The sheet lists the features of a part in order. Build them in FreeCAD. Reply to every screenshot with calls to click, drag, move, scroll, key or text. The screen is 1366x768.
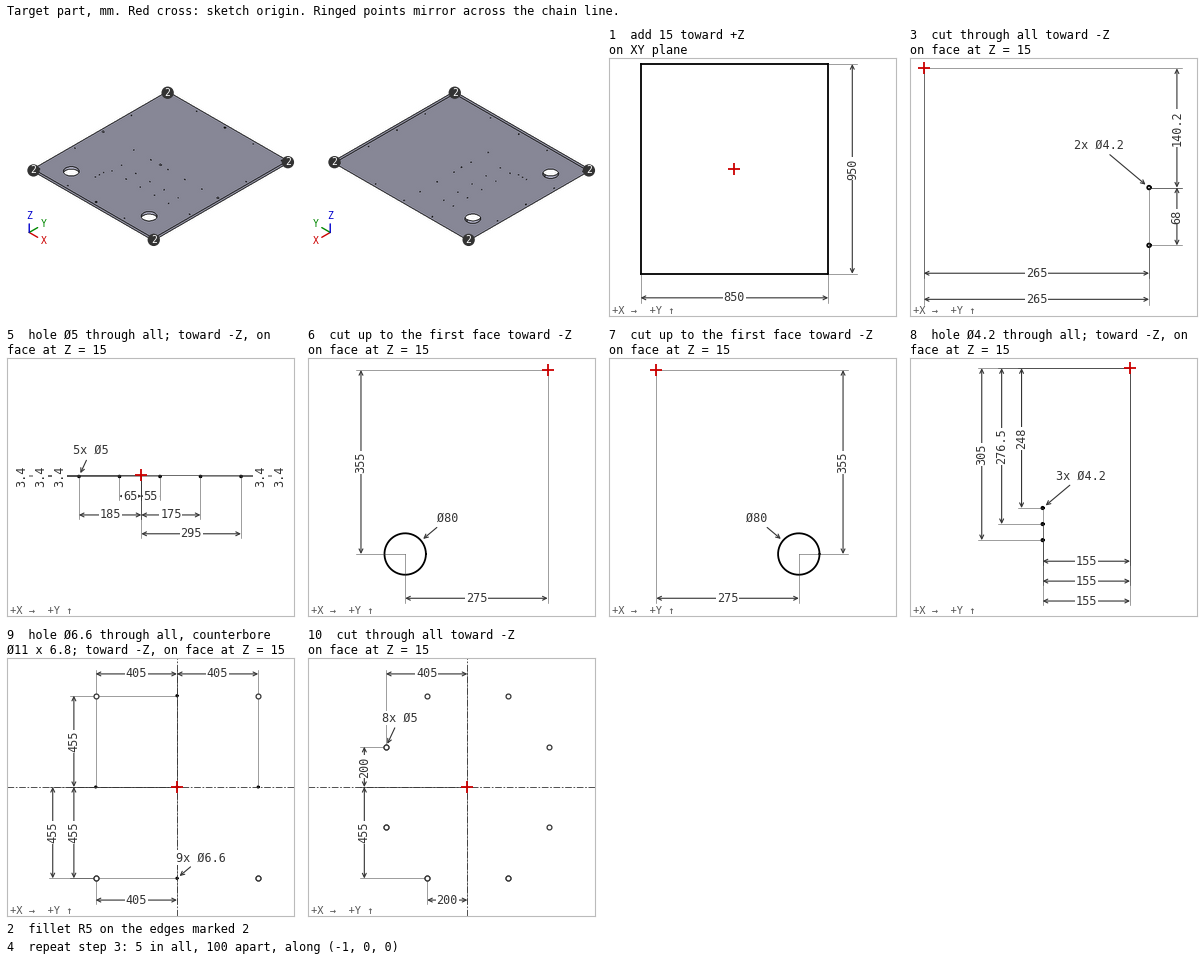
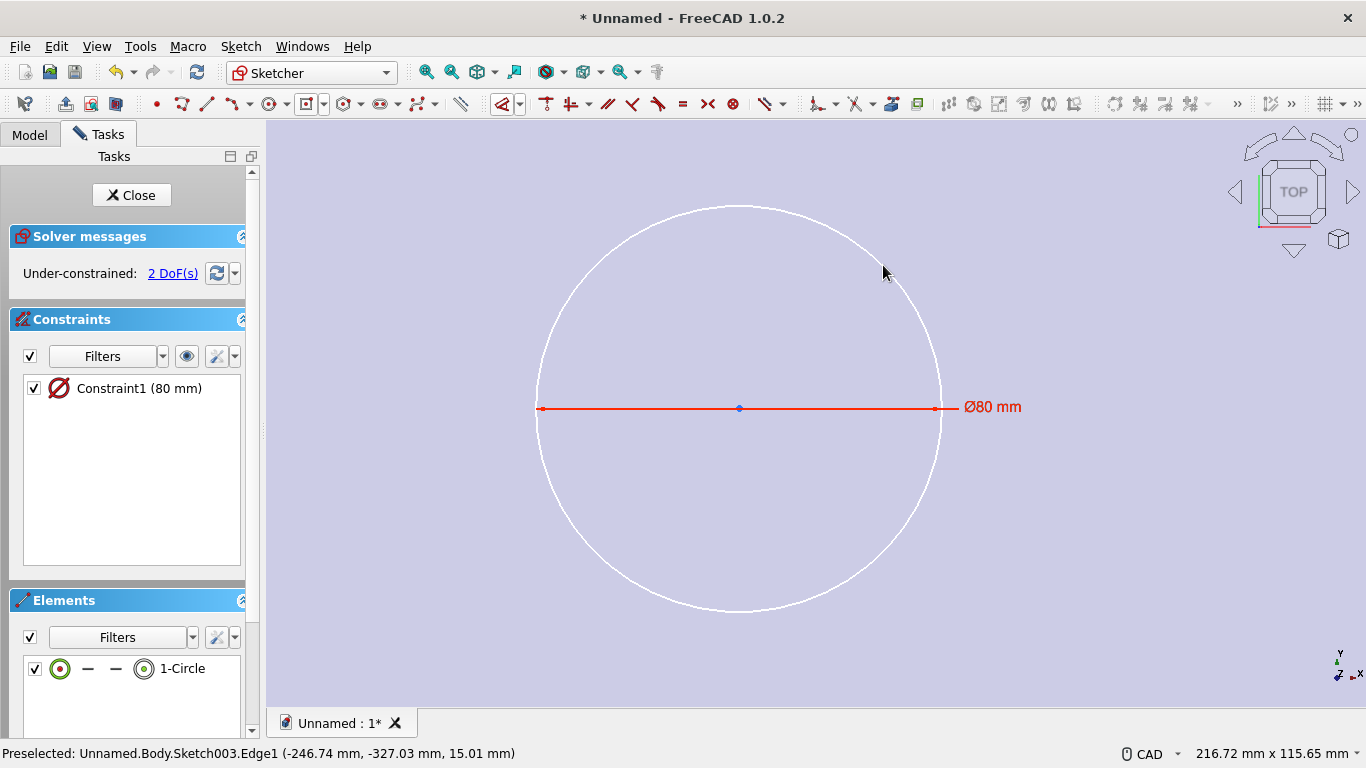
click(739, 409)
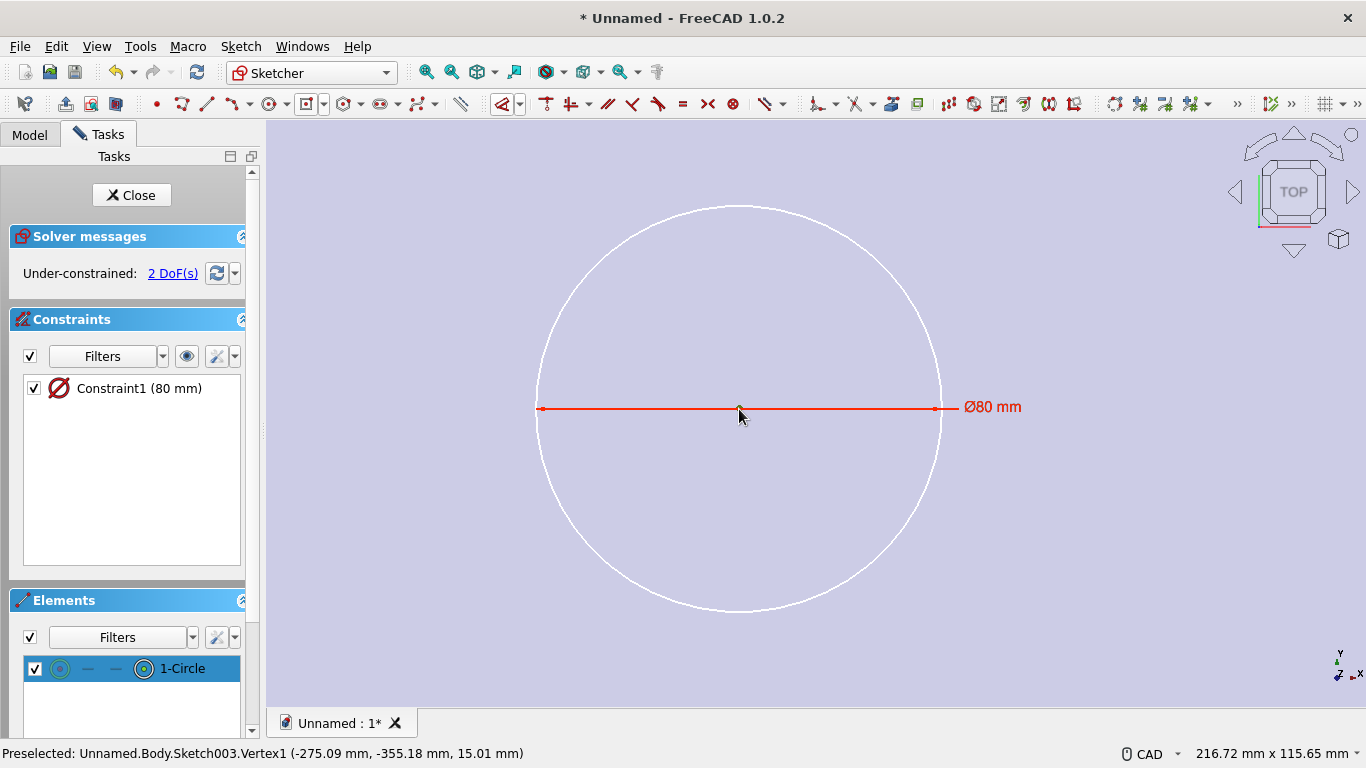
click(520, 104)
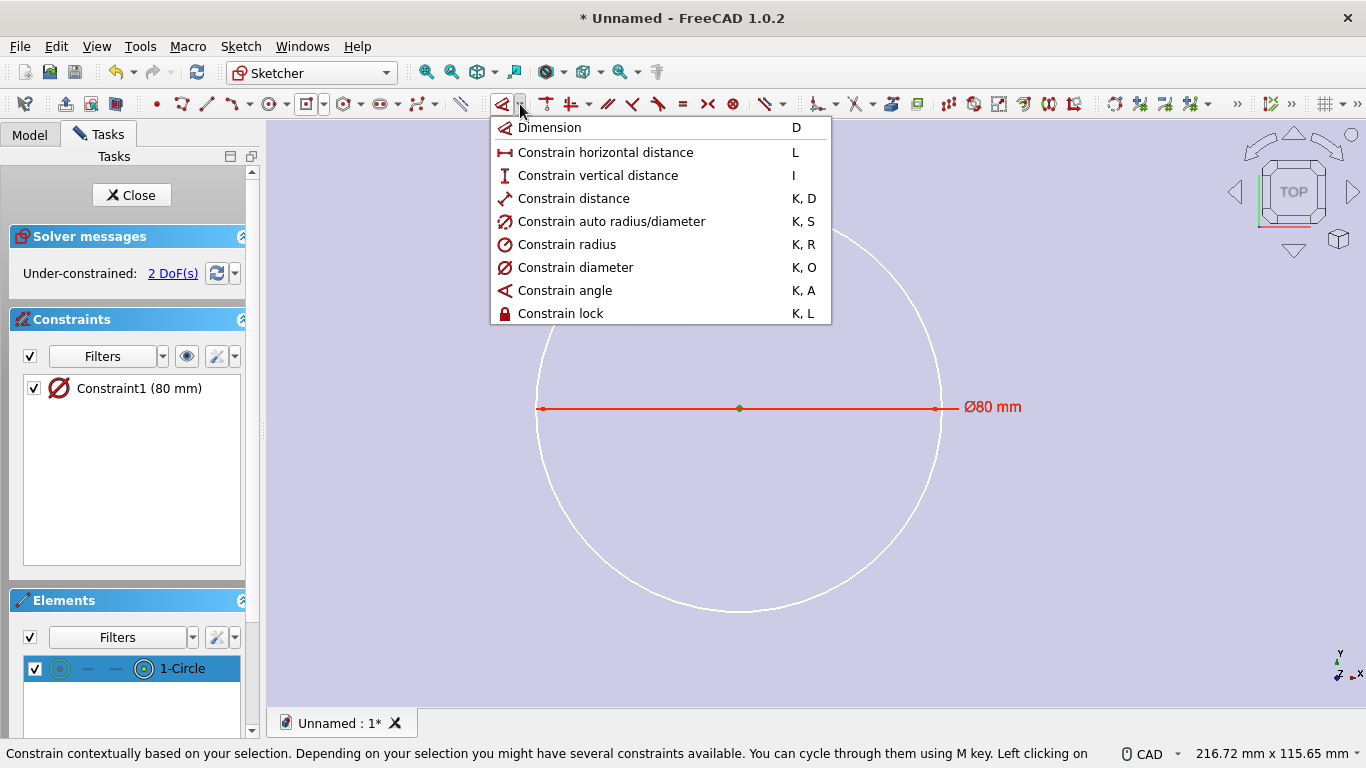
click(661, 152)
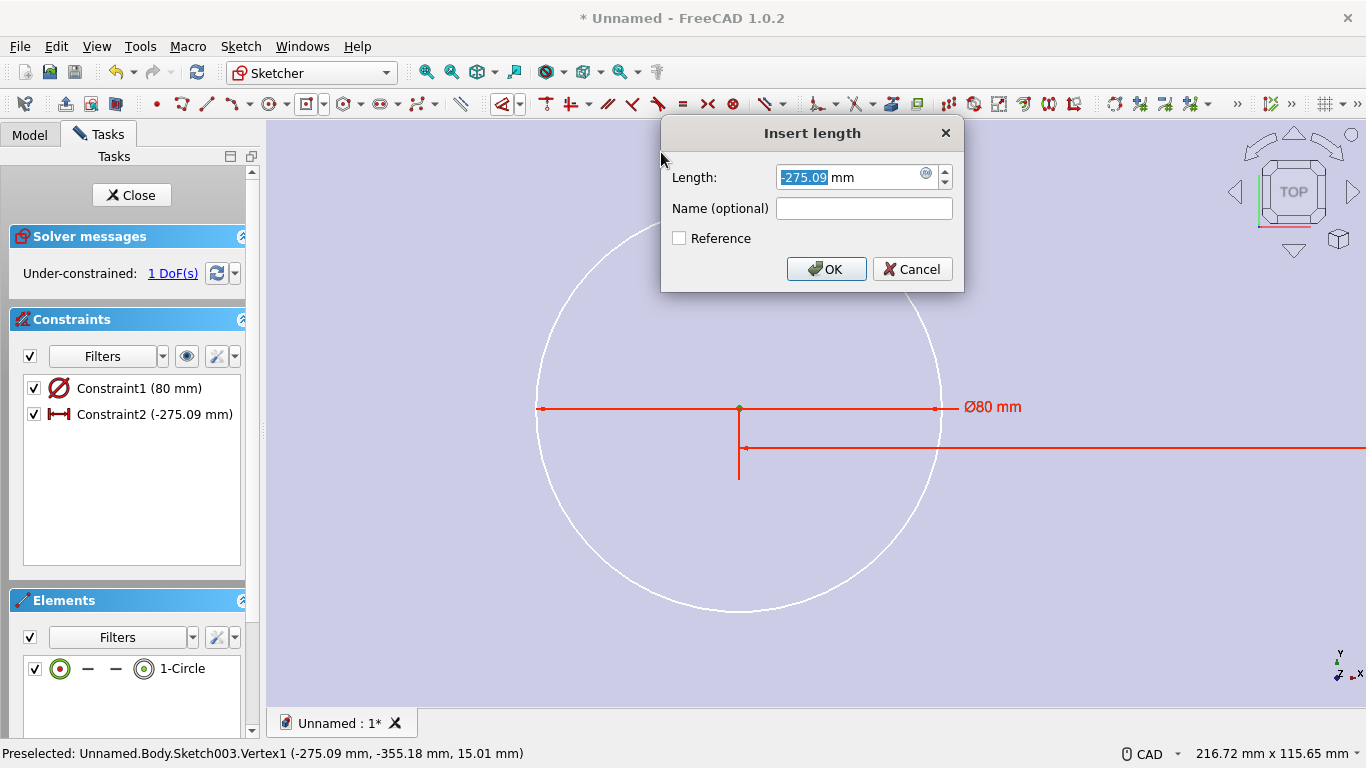
text(-275)
key(Return)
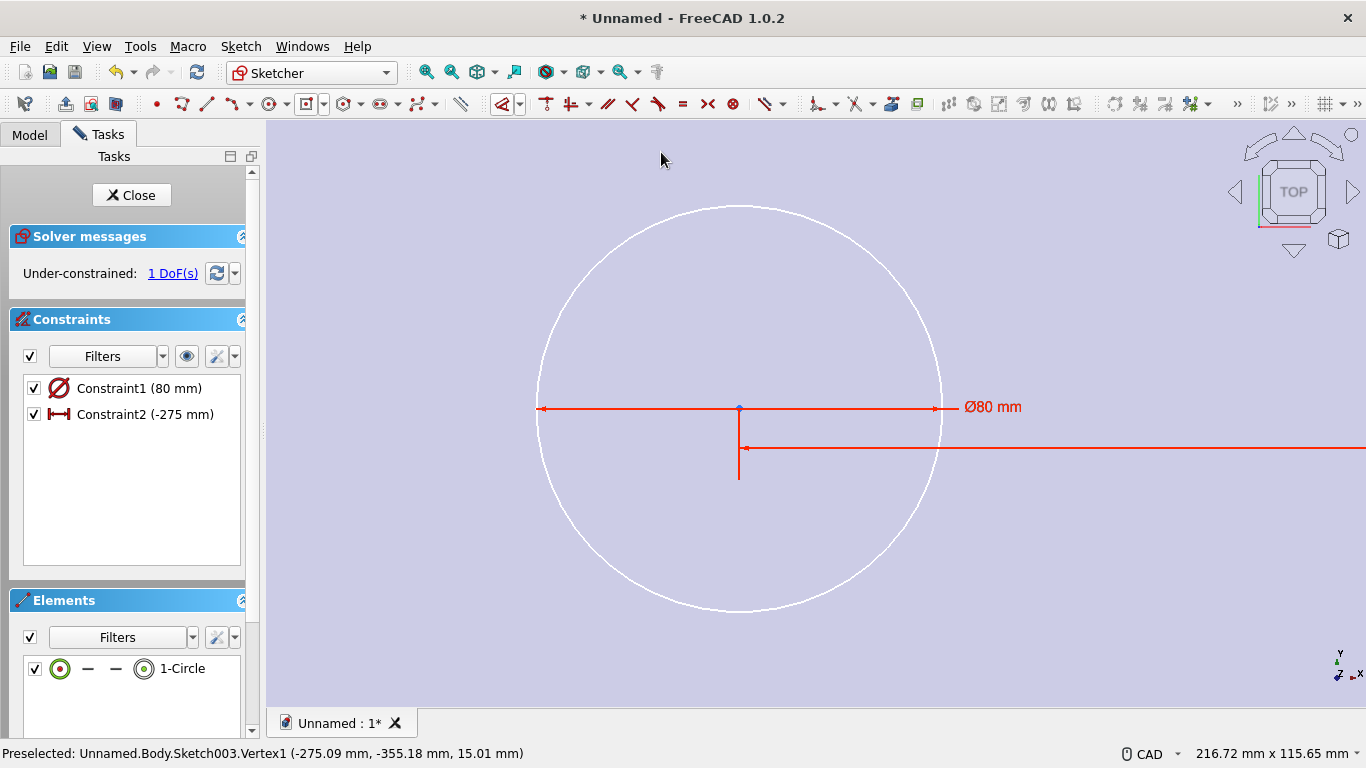
click(739, 409)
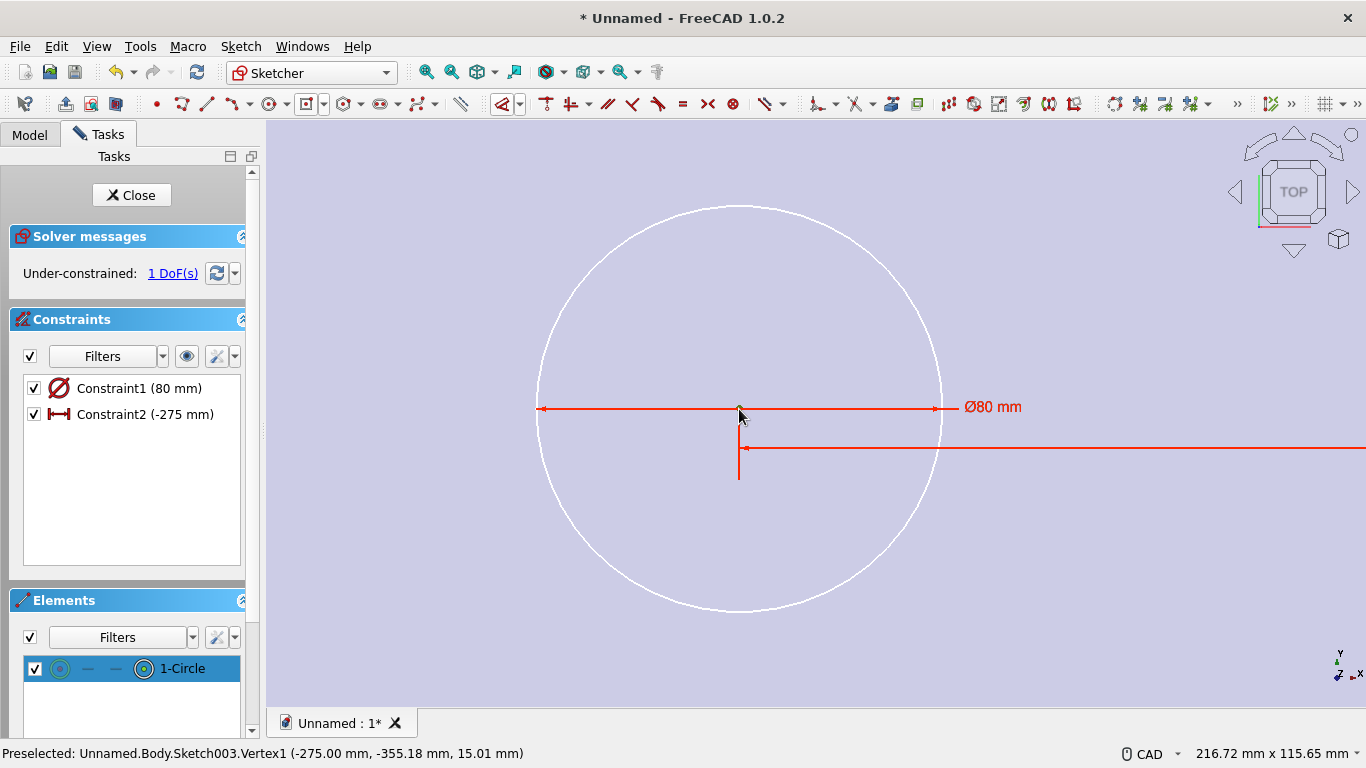
click(520, 104)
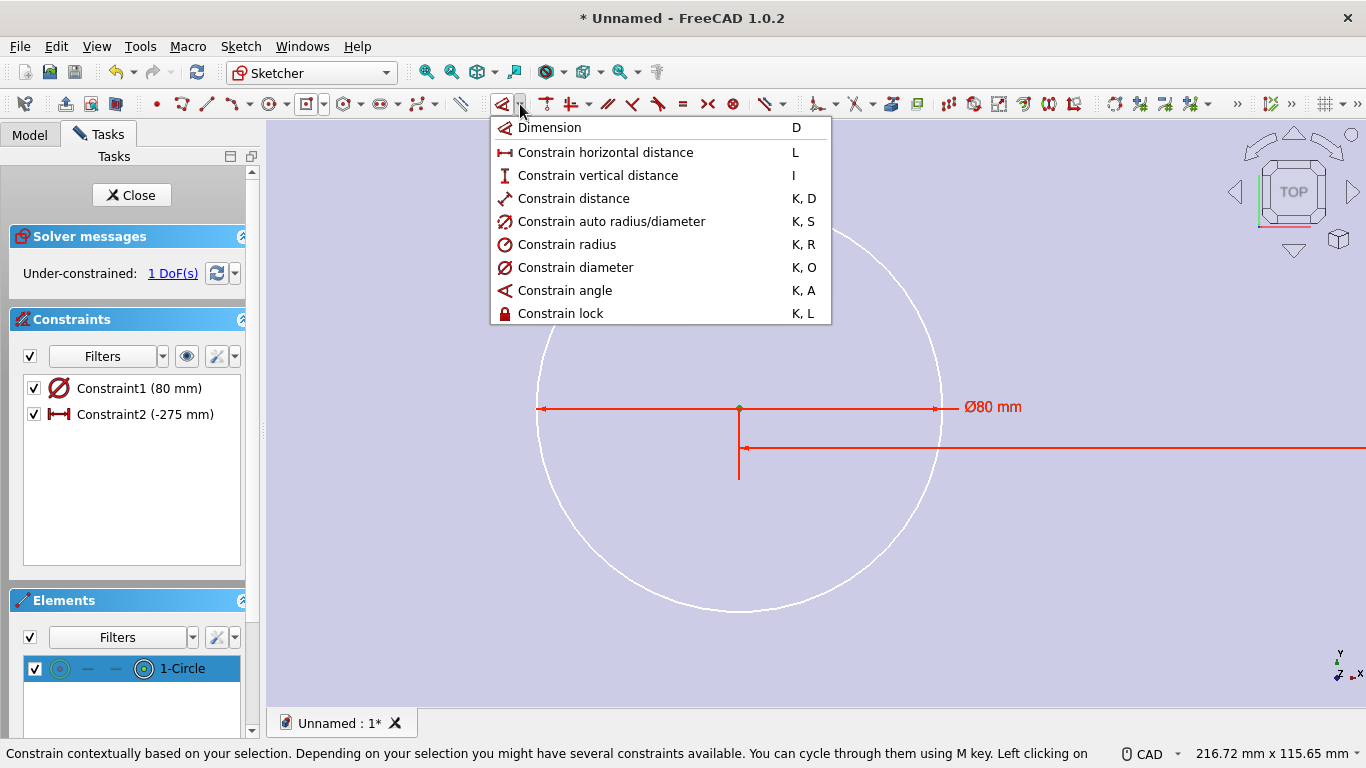
click(661, 176)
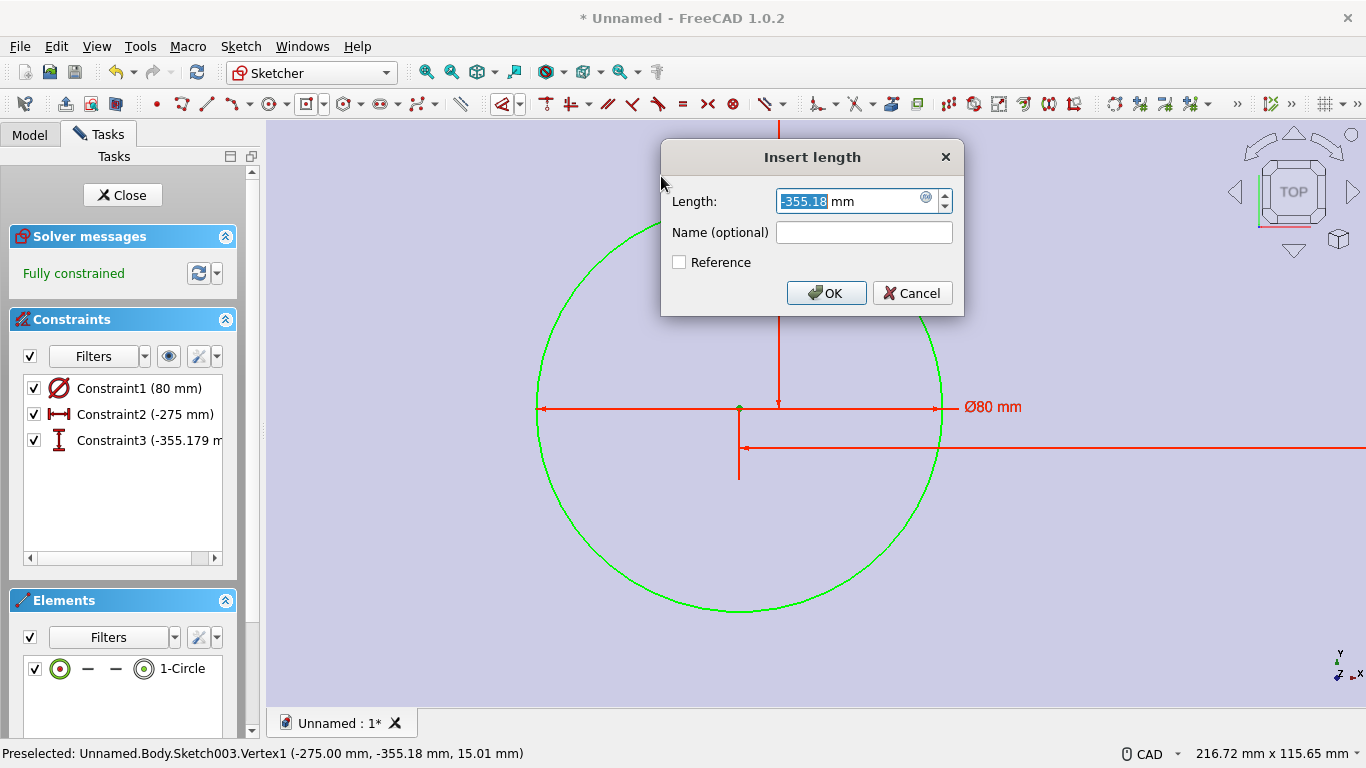
text(-355)
key(Return)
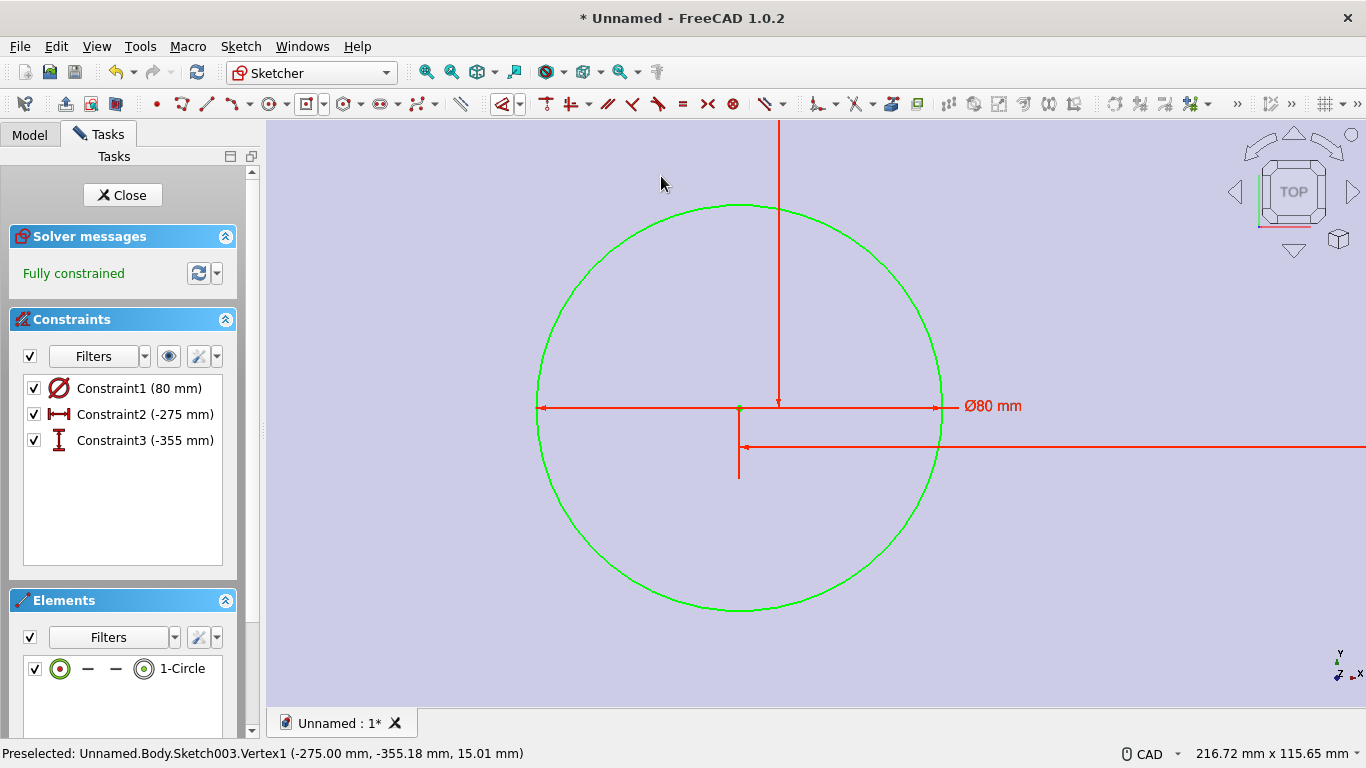
click(123, 195)